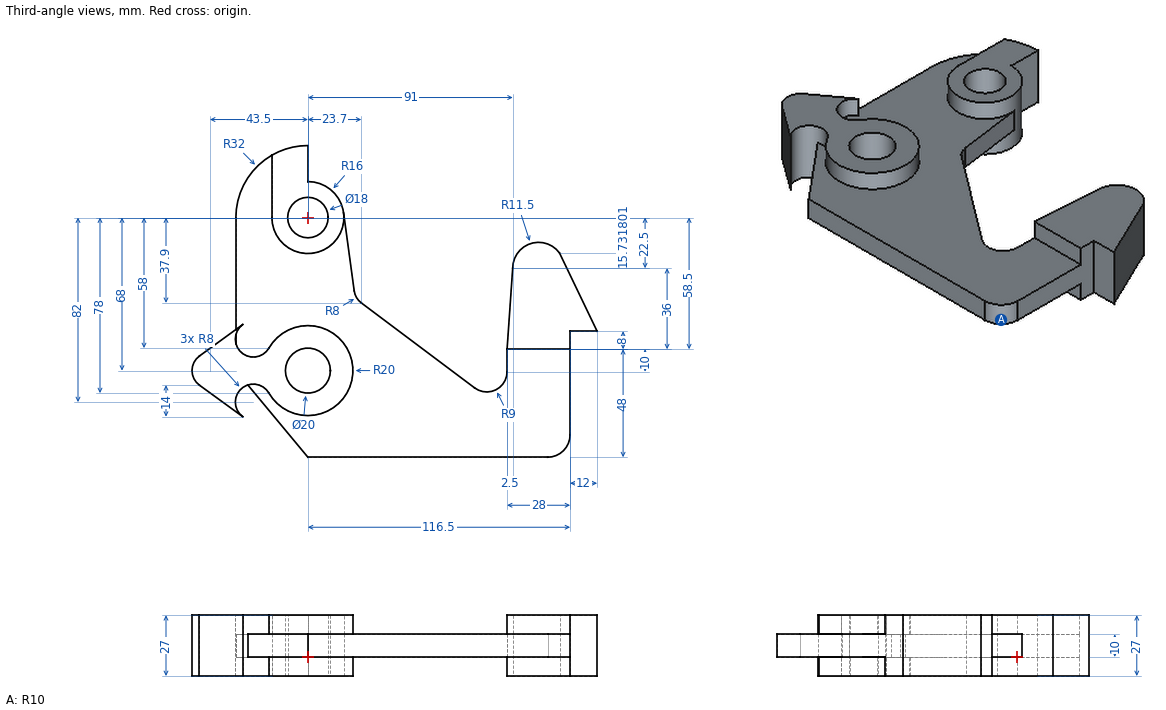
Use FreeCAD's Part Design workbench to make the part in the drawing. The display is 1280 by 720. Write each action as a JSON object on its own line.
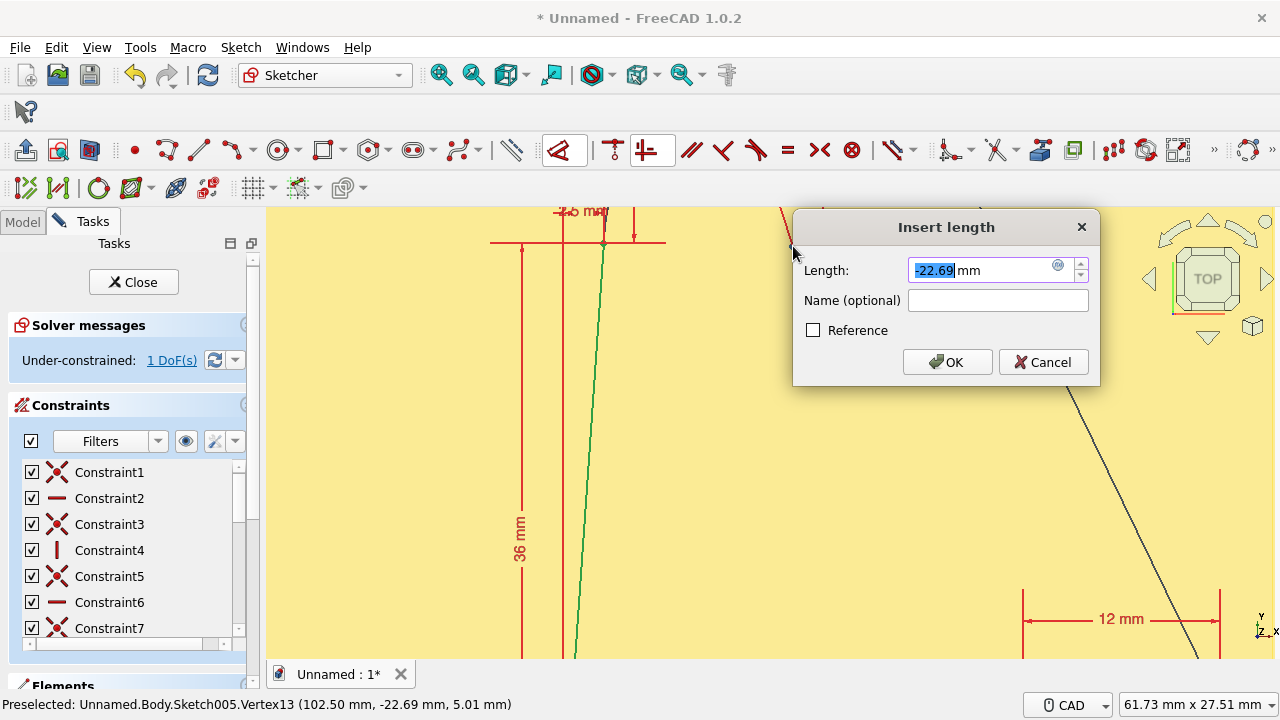
{"action": "type", "text": "-22.5"}
{"action": "key", "text": "Return"}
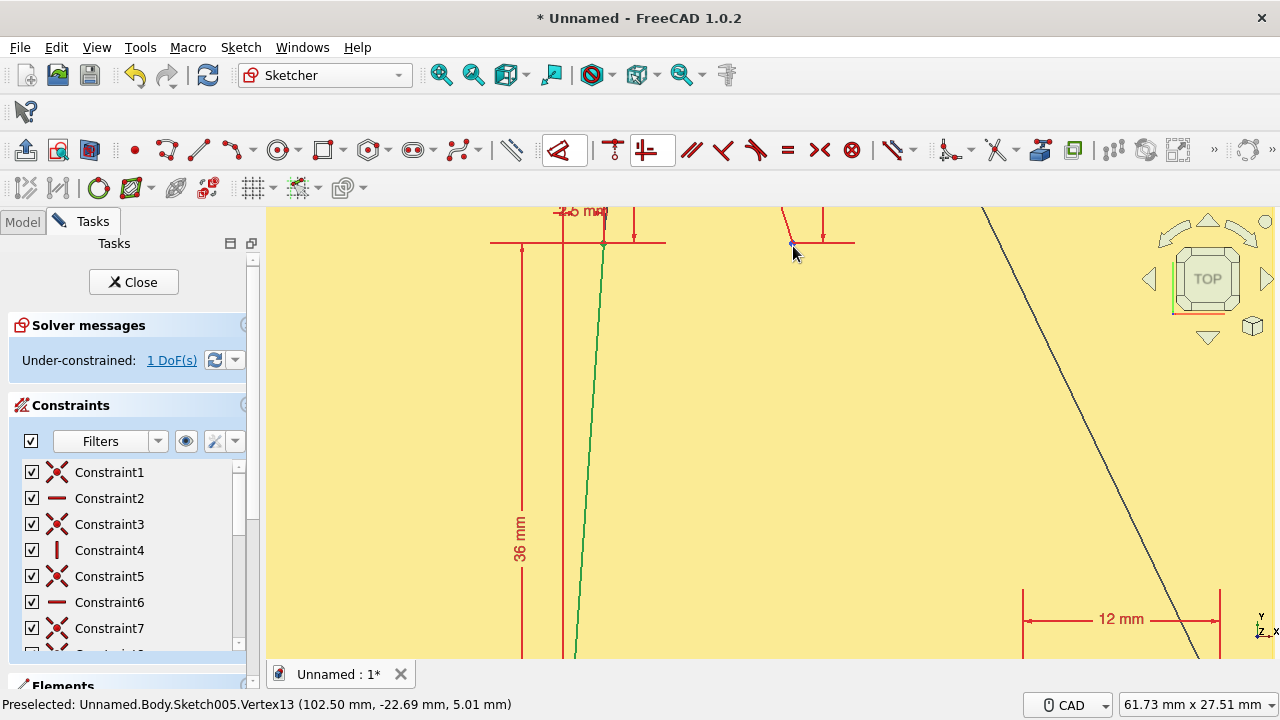
{"action": "scroll", "coordinate": [596, 424], "scroll_direction": "down", "scroll_amount": 5}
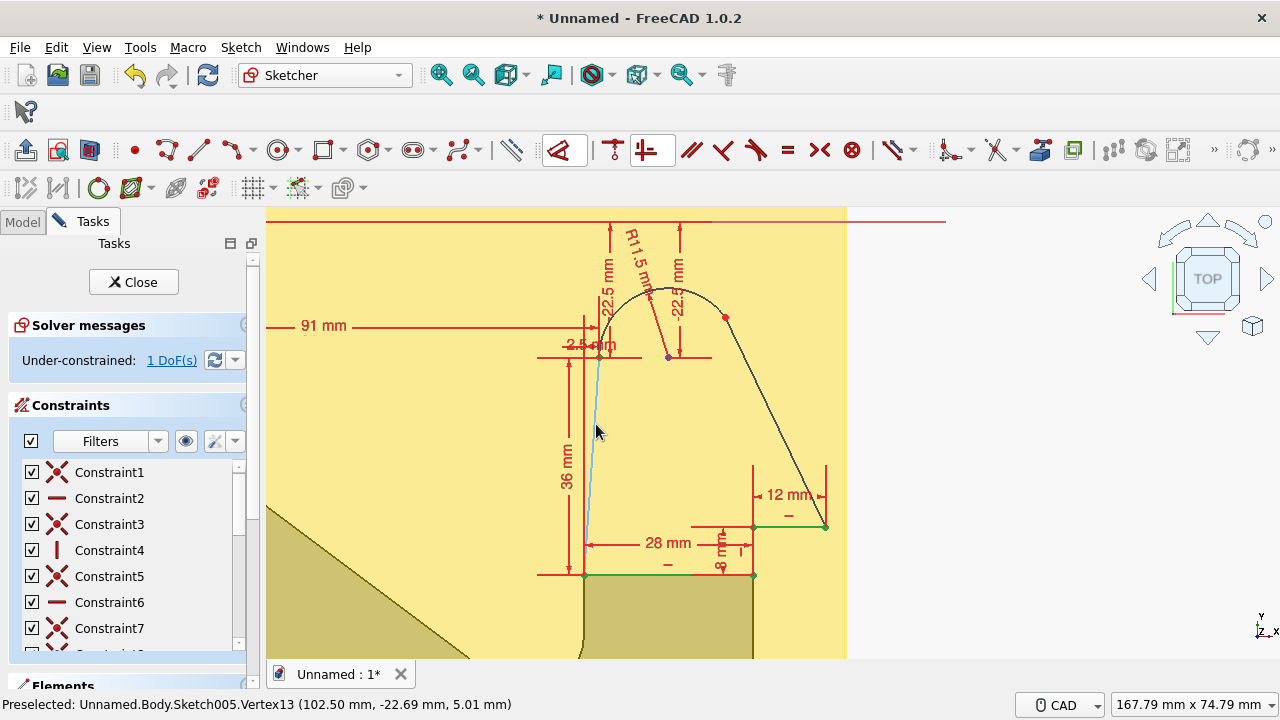
{"action": "left_click", "coordinate": [725, 318]}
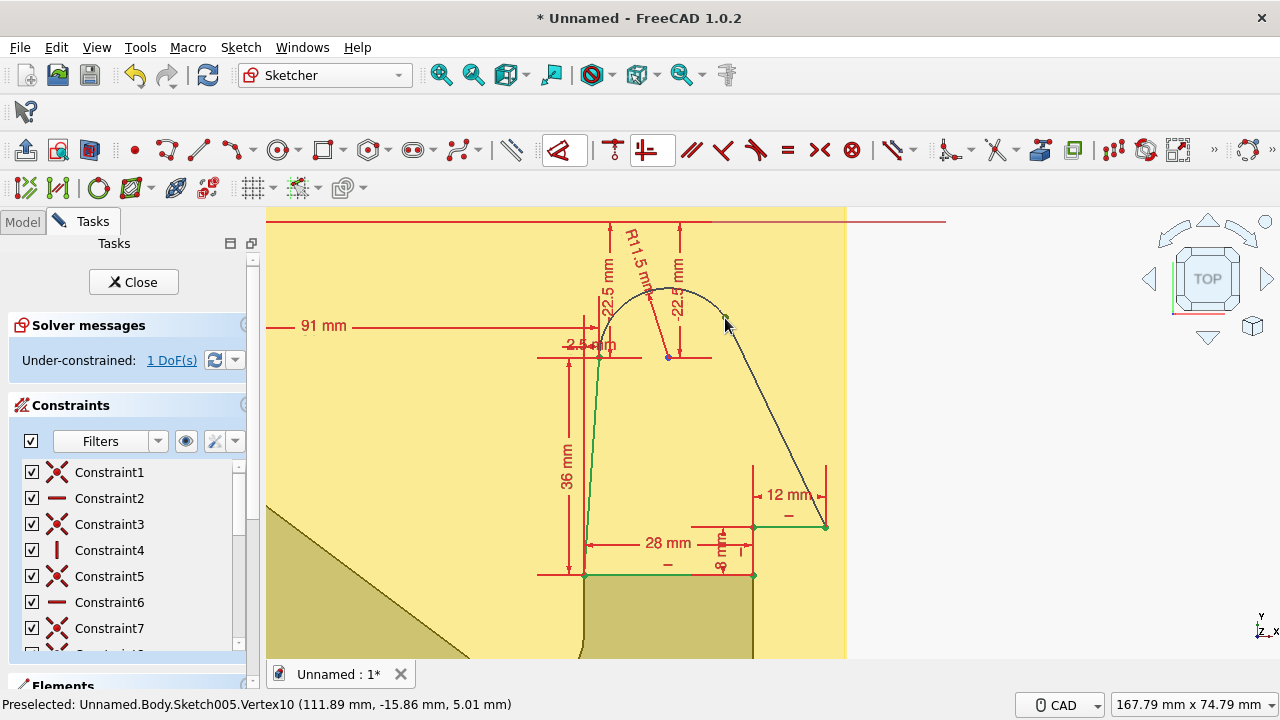
{"action": "key", "text": "i"}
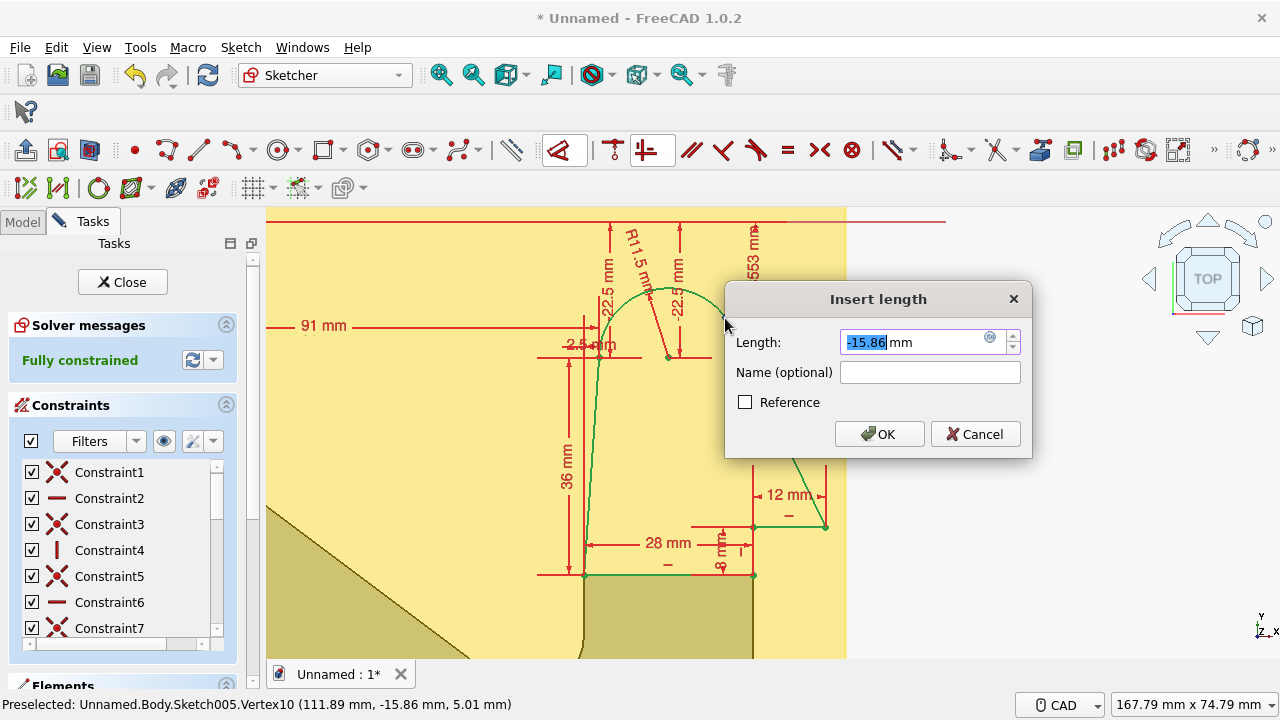
{"action": "type", "text": "-15.731801"}
{"action": "key", "text": "Return"}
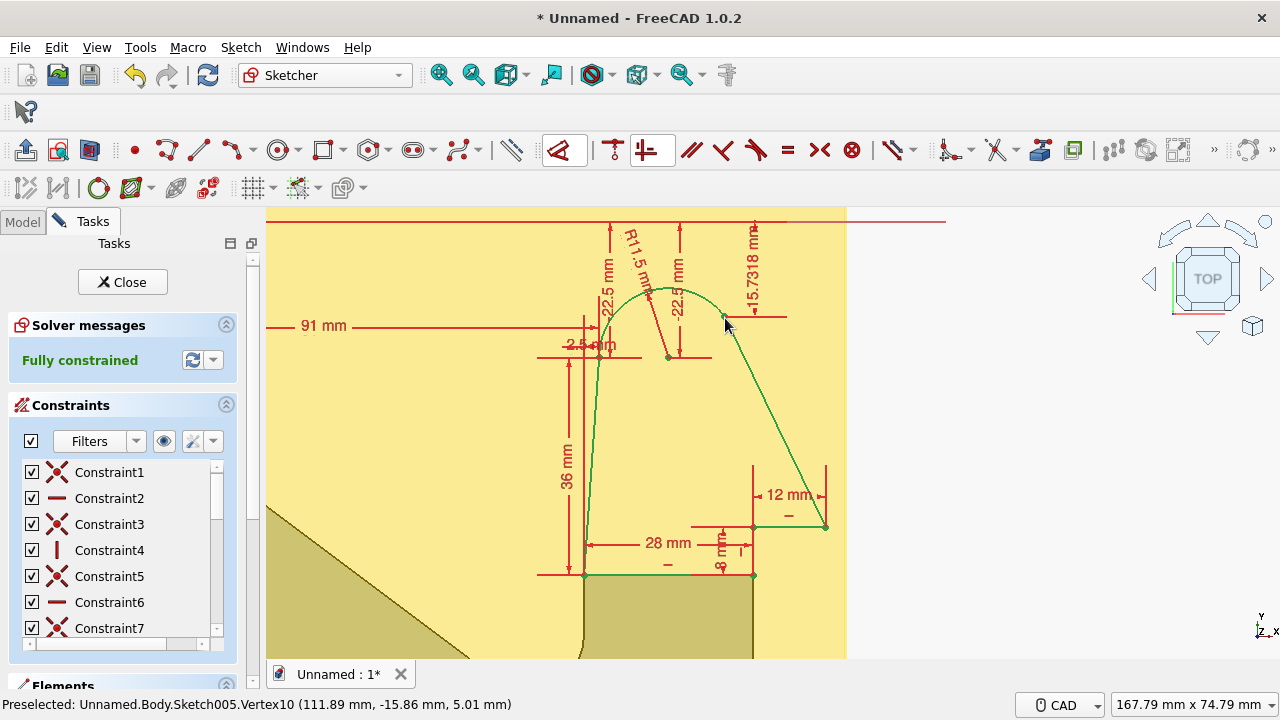
{"action": "left_click", "coordinate": [123, 282]}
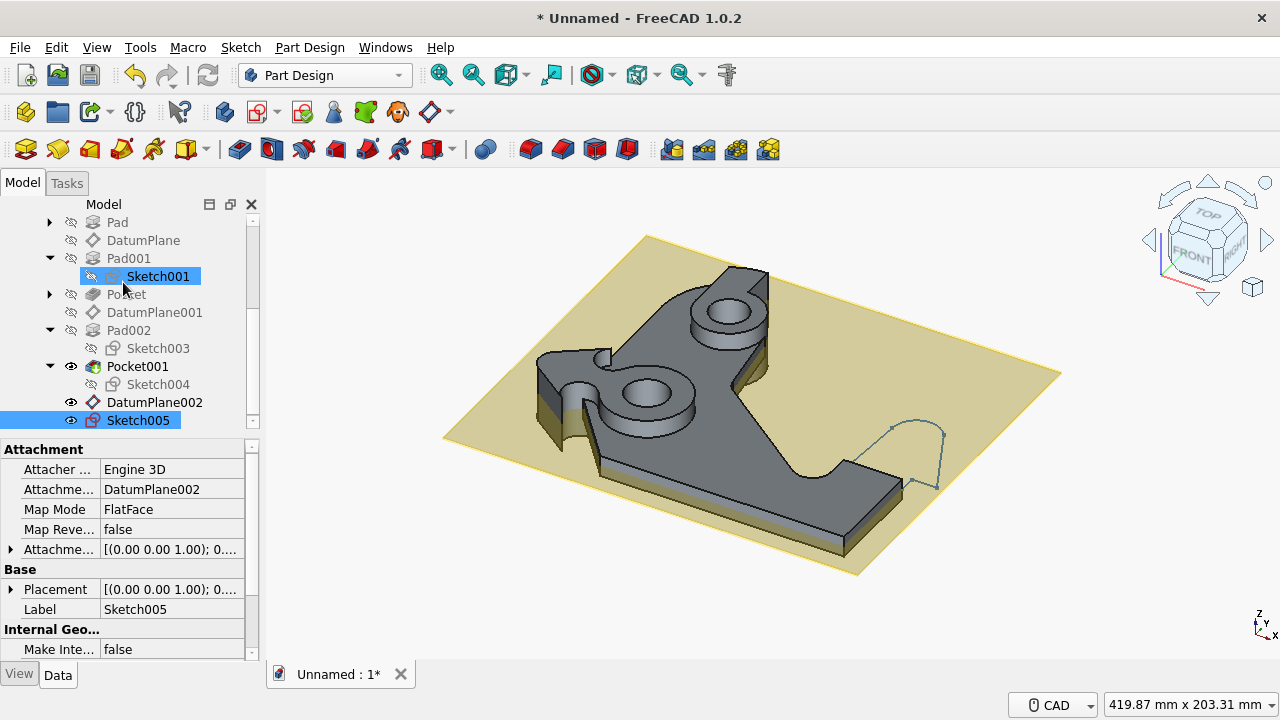
{"action": "left_click", "coordinate": [26, 150]}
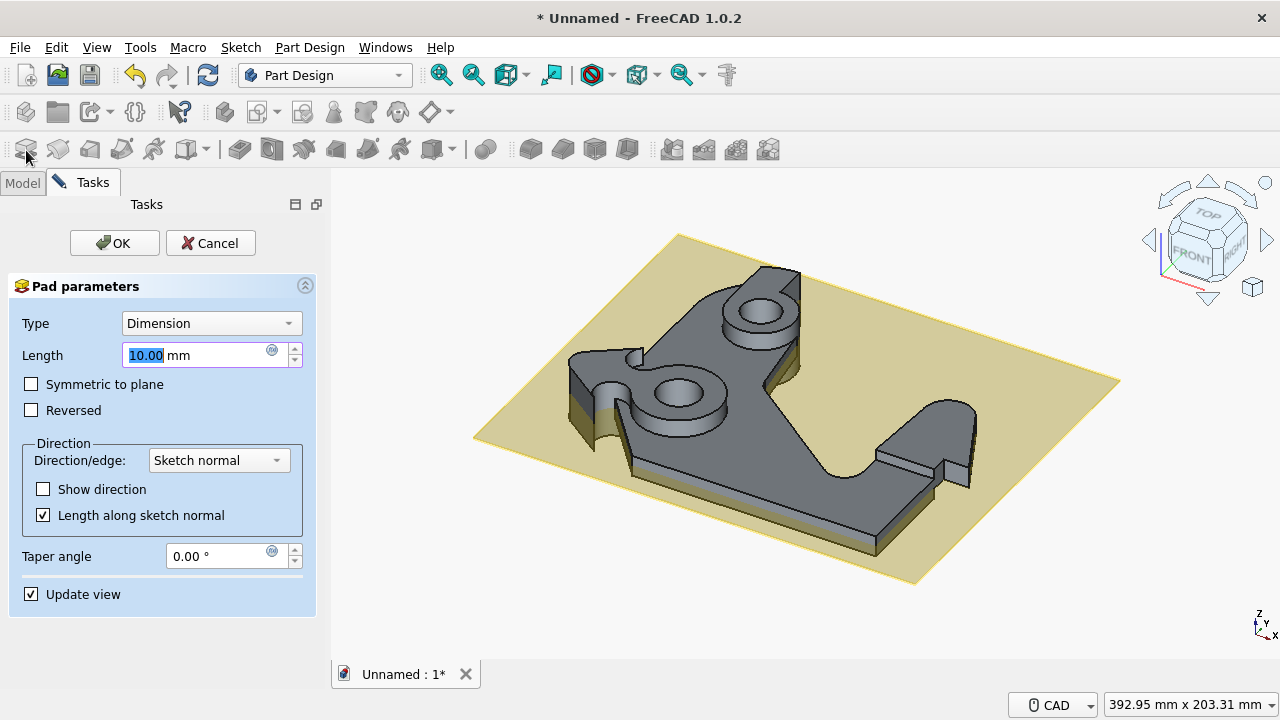
{"action": "type", "text": "27"}
{"action": "key", "text": "Tab"}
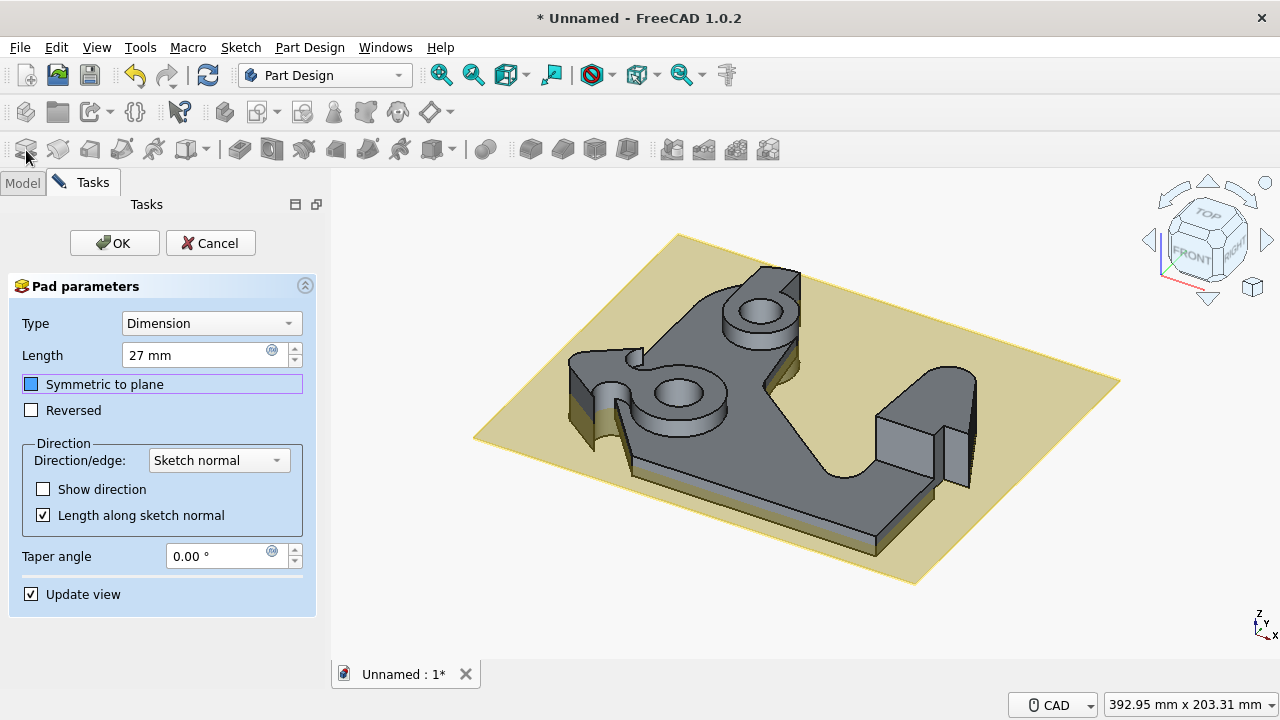
{"action": "left_click", "coordinate": [30, 384]}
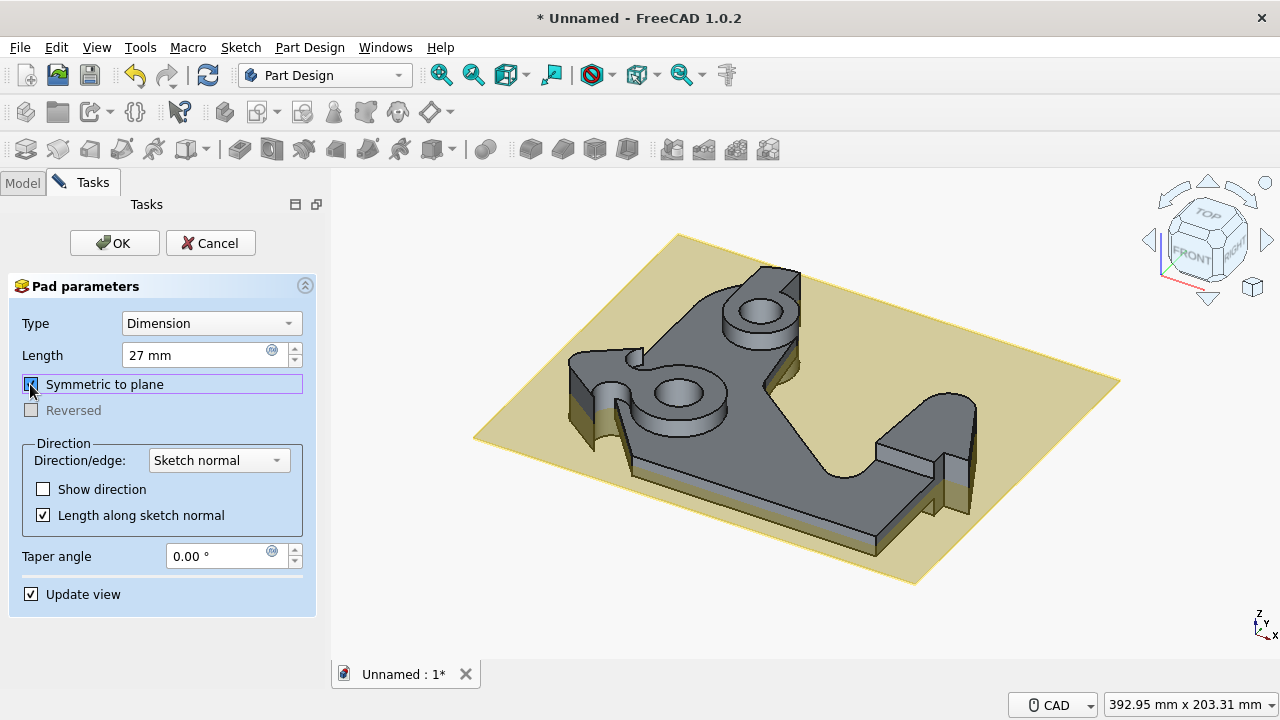
{"action": "left_click", "coordinate": [115, 243]}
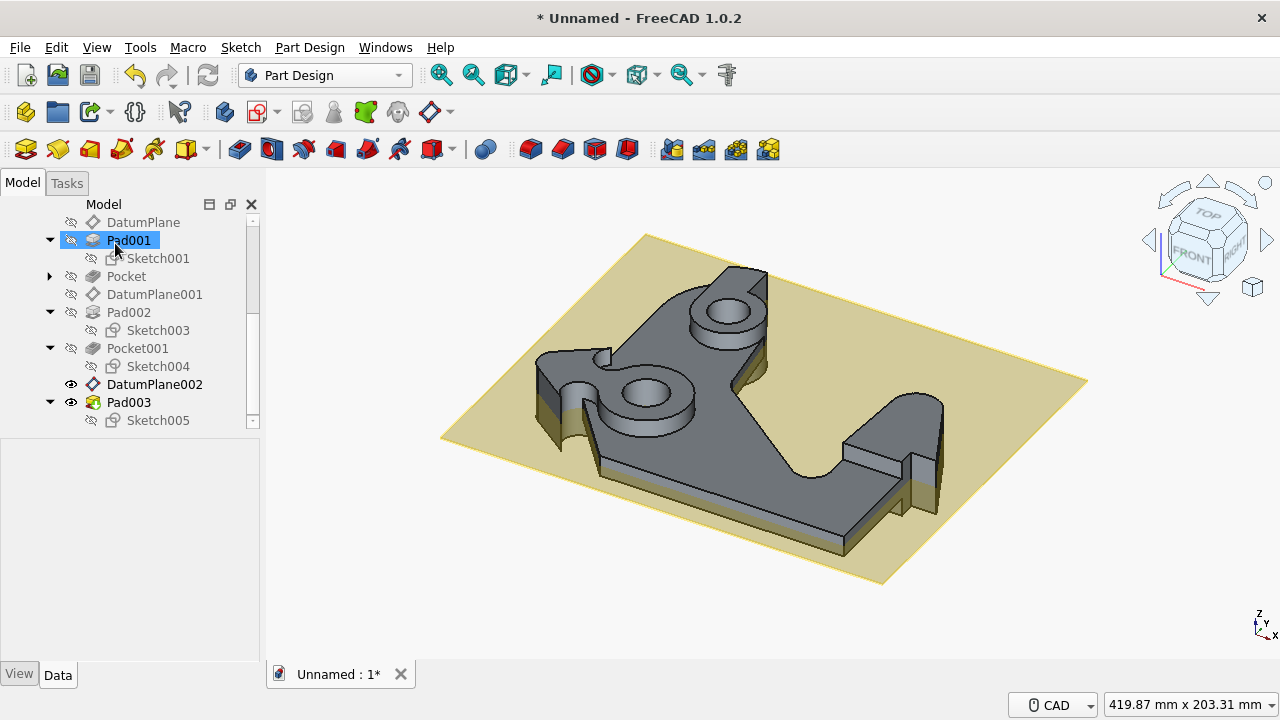
{"action": "left_click", "coordinate": [116, 384]}
{"action": "key", "text": "space"}